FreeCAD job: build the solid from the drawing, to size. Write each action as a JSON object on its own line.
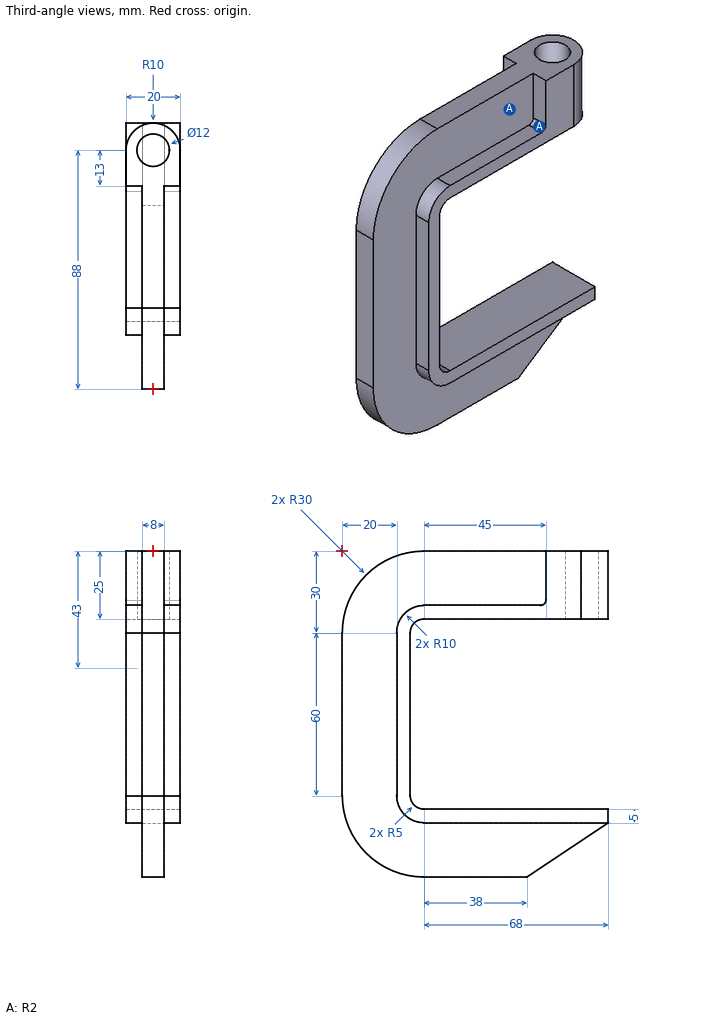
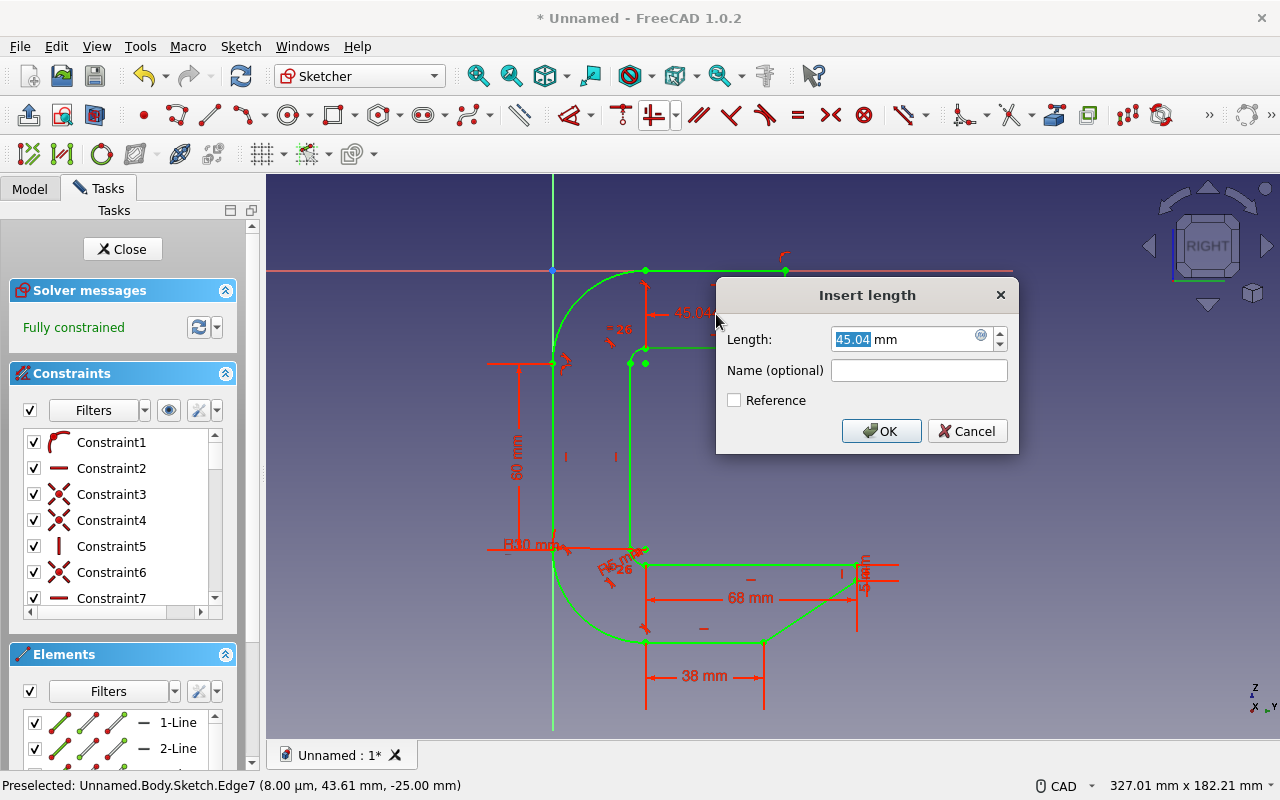
{"action": "type", "text": "45"}
{"action": "key", "text": "Return"}
{"action": "key", "text": "Escape"}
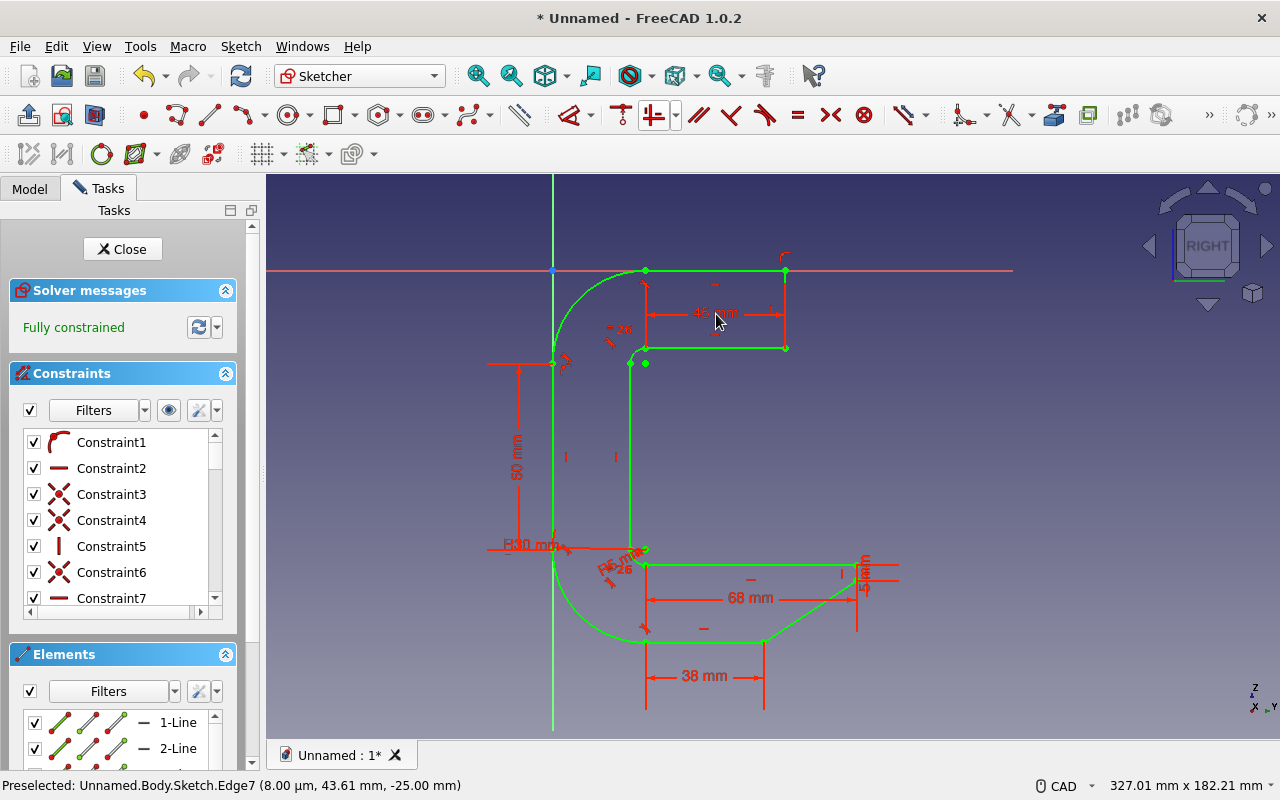
{"action": "left_click", "coordinate": [123, 249]}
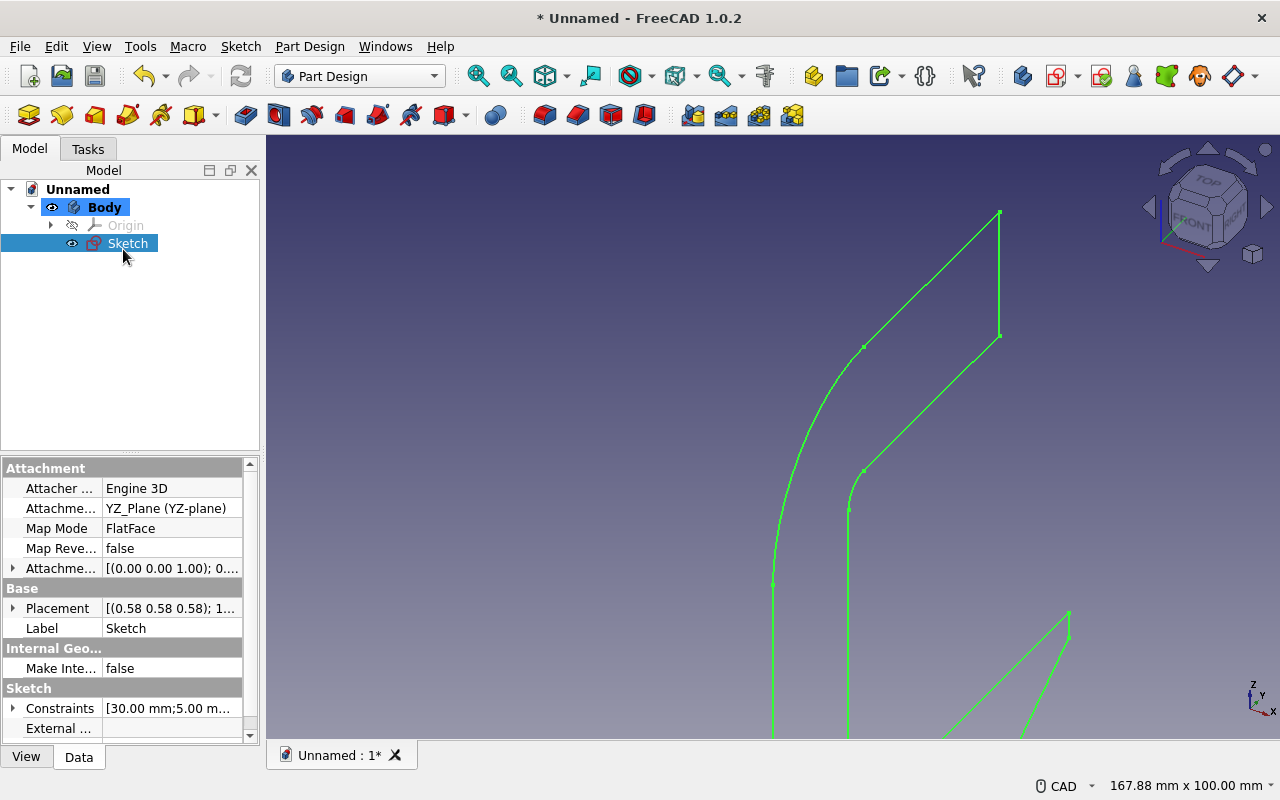
{"action": "left_click", "coordinate": [29, 116]}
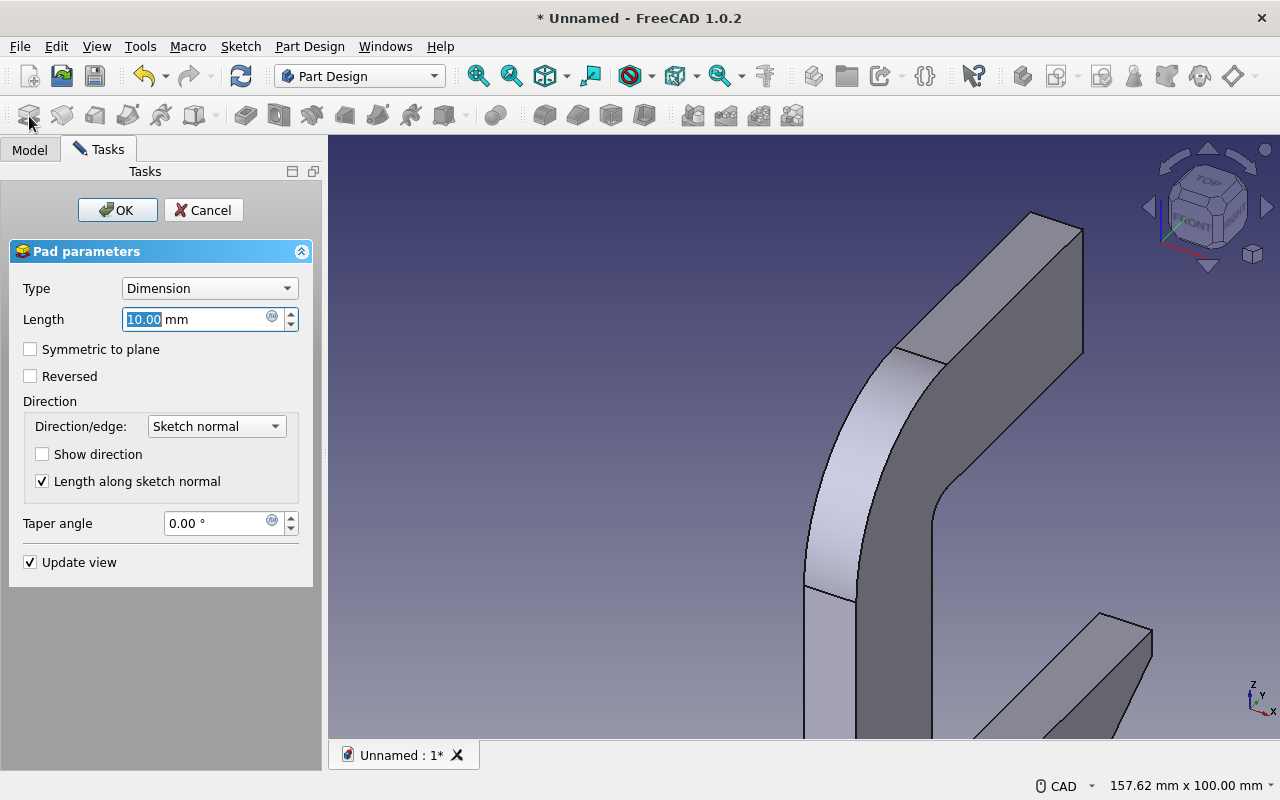
{"action": "type", "text": "8"}
{"action": "key", "text": "Tab"}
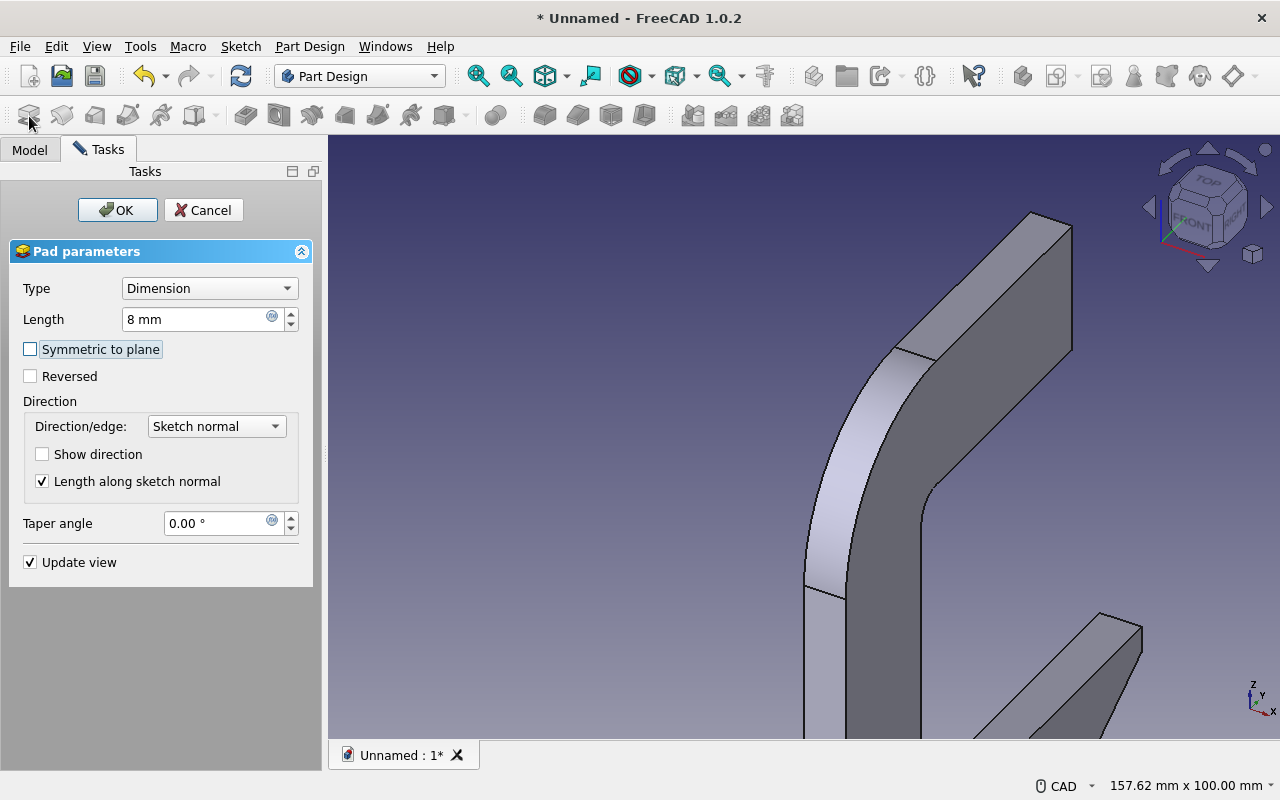
{"action": "left_click", "coordinate": [31, 349]}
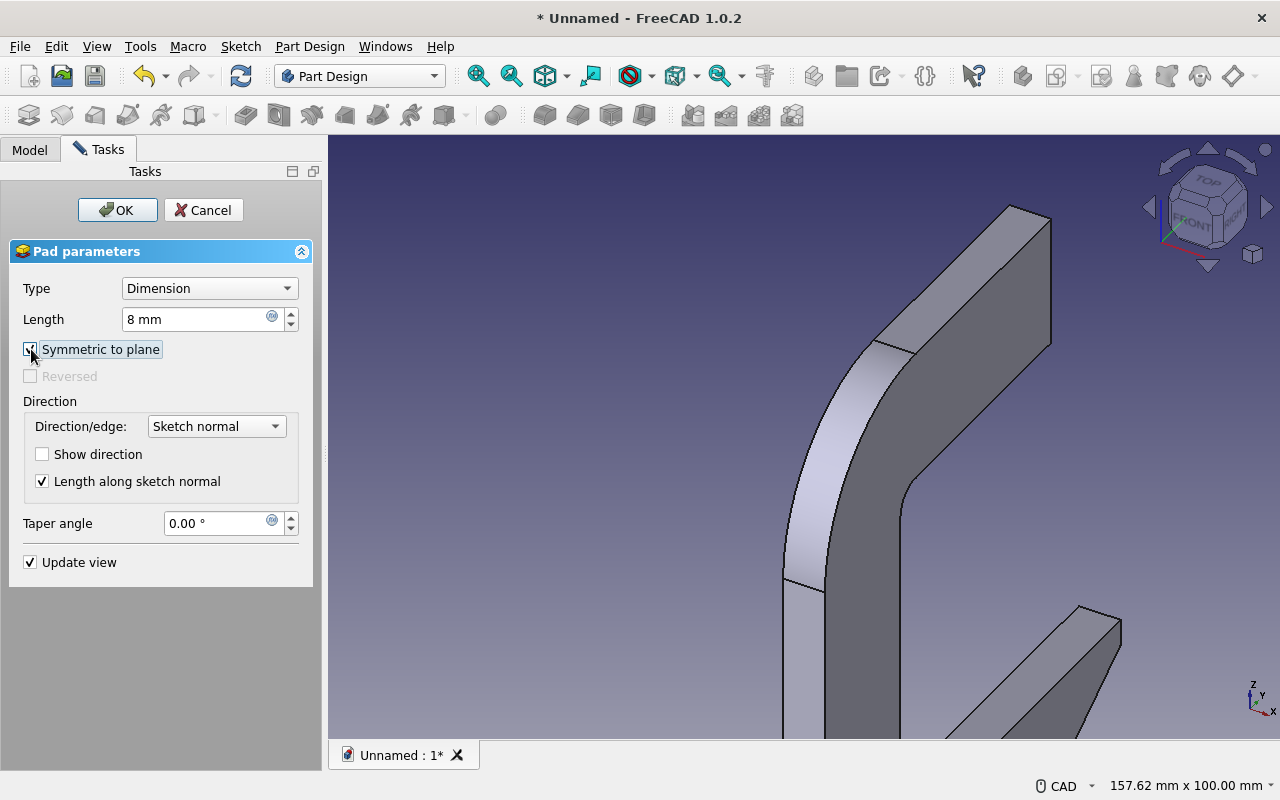
{"action": "left_click", "coordinate": [118, 210]}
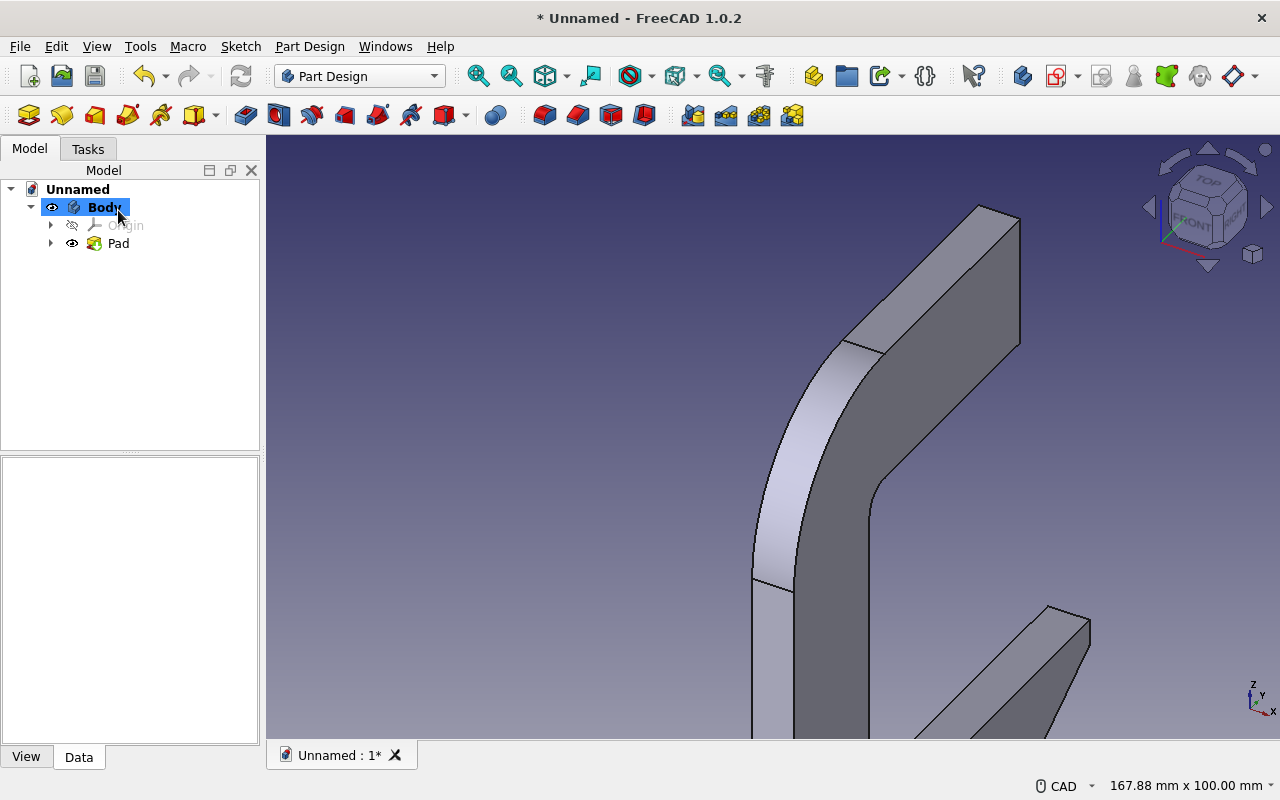
{"action": "key", "text": "v f"}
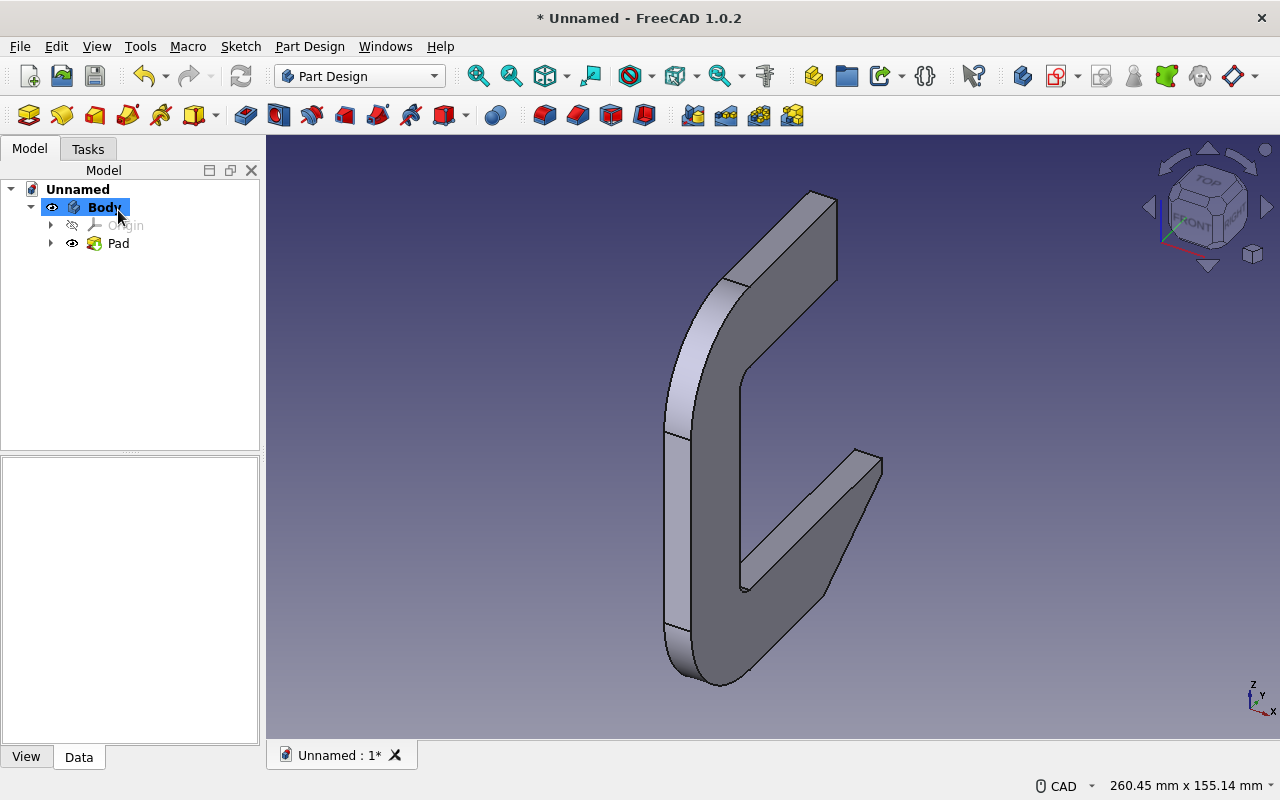
{"action": "left_click", "coordinate": [1056, 76]}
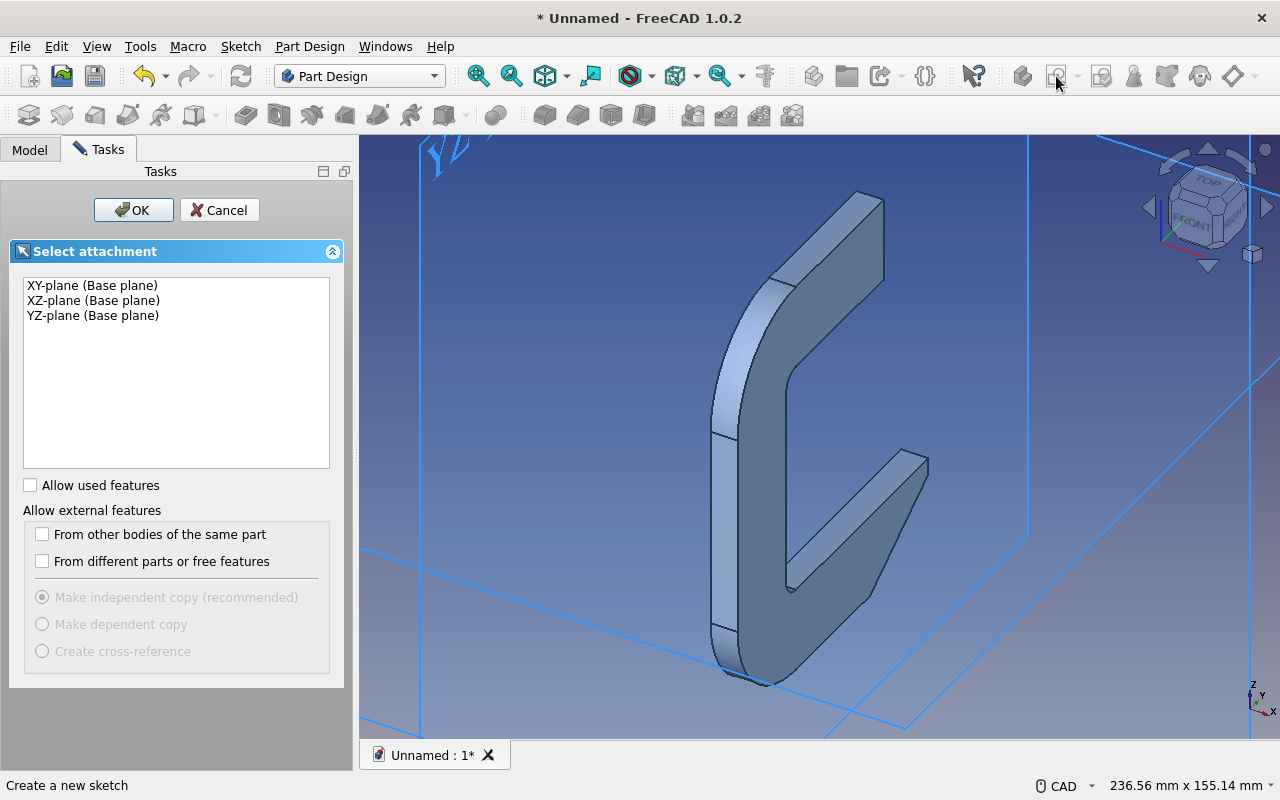
{"action": "left_click", "coordinate": [84, 316]}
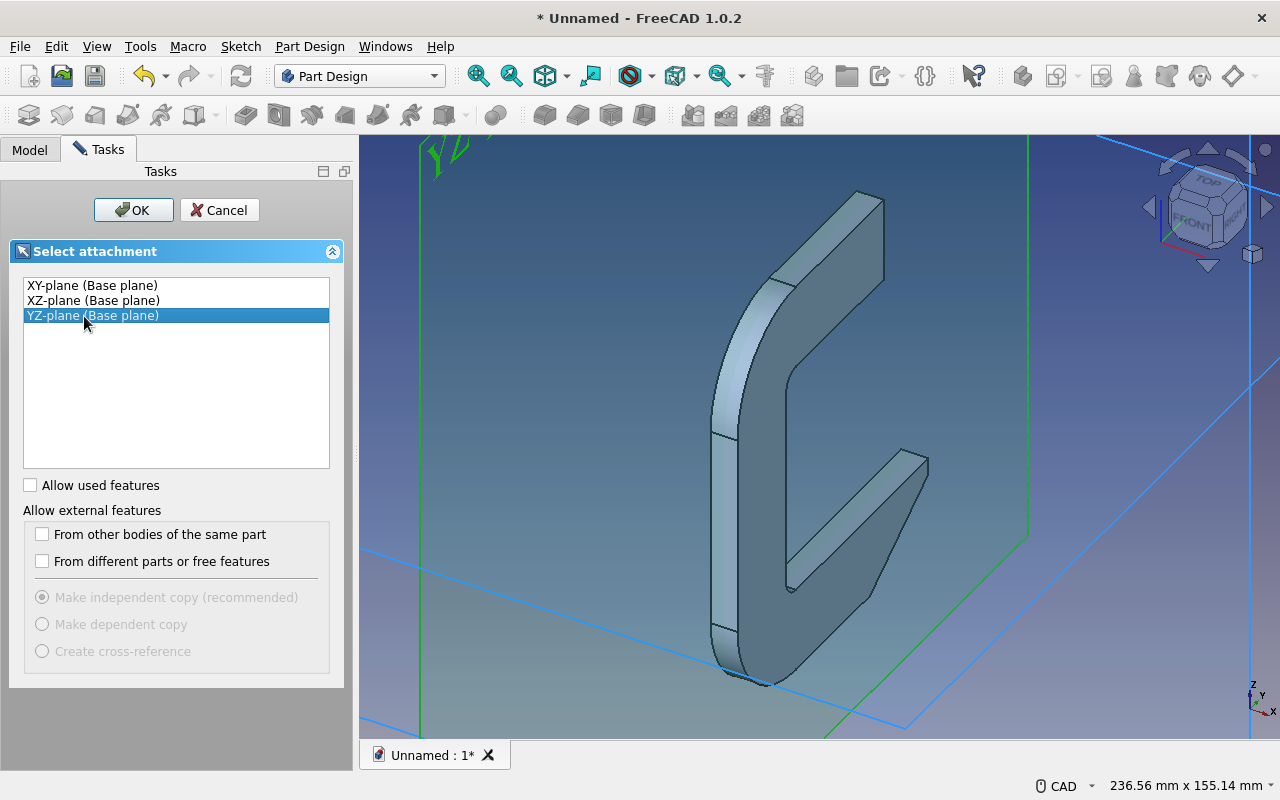
{"action": "left_click", "coordinate": [134, 210]}